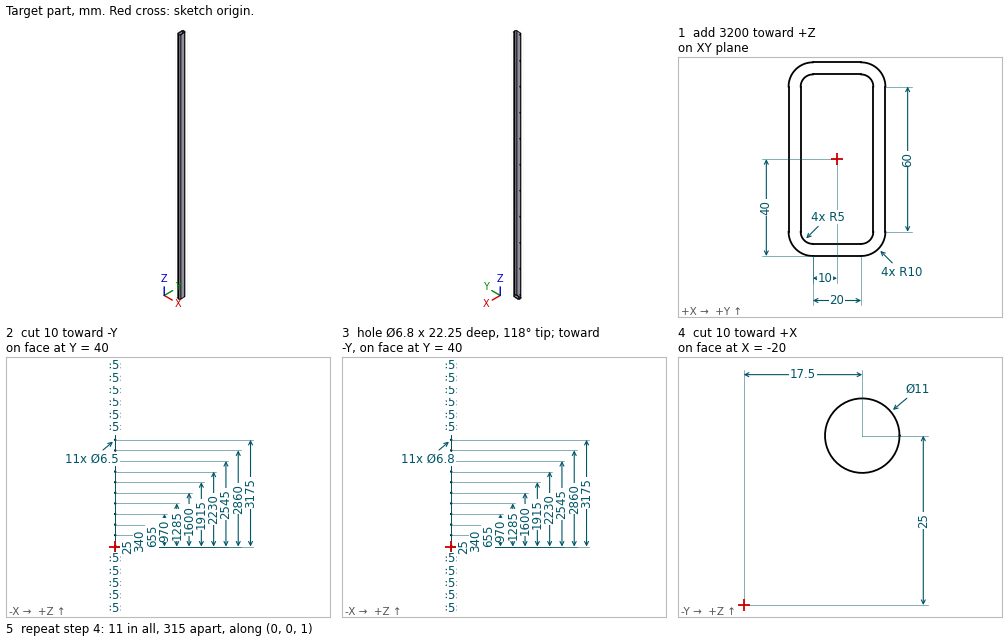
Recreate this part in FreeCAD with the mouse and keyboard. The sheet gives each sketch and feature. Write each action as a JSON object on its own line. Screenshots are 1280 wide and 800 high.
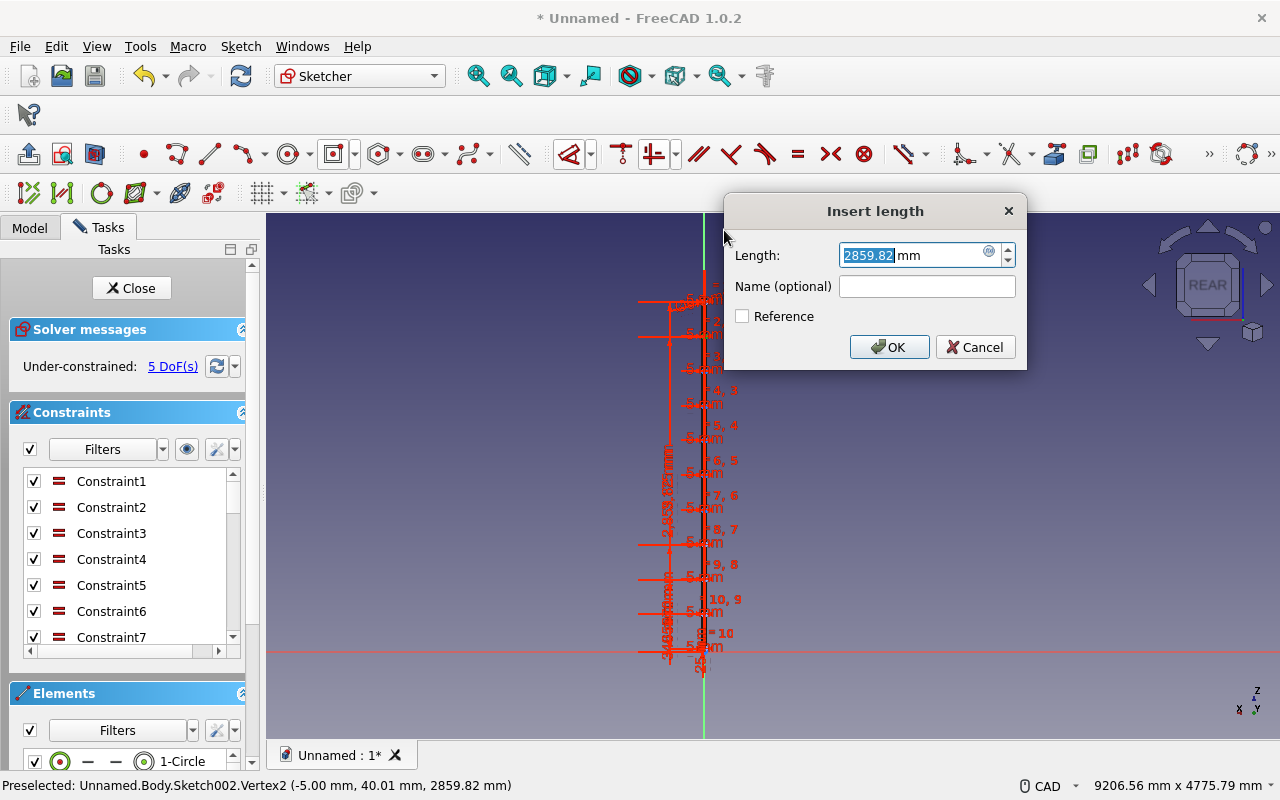
{"action": "type", "text": "2860"}
{"action": "key", "text": "Return"}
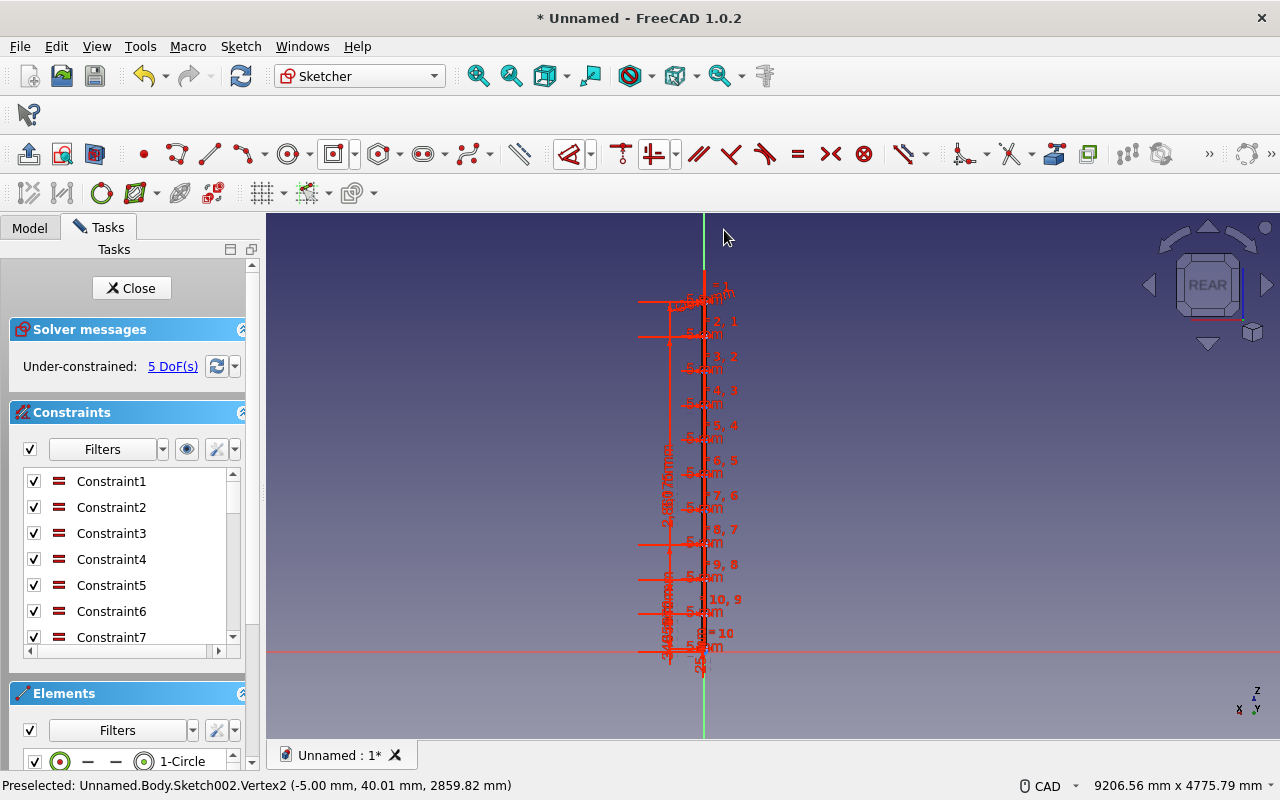
{"action": "left_click", "coordinate": [705, 371]}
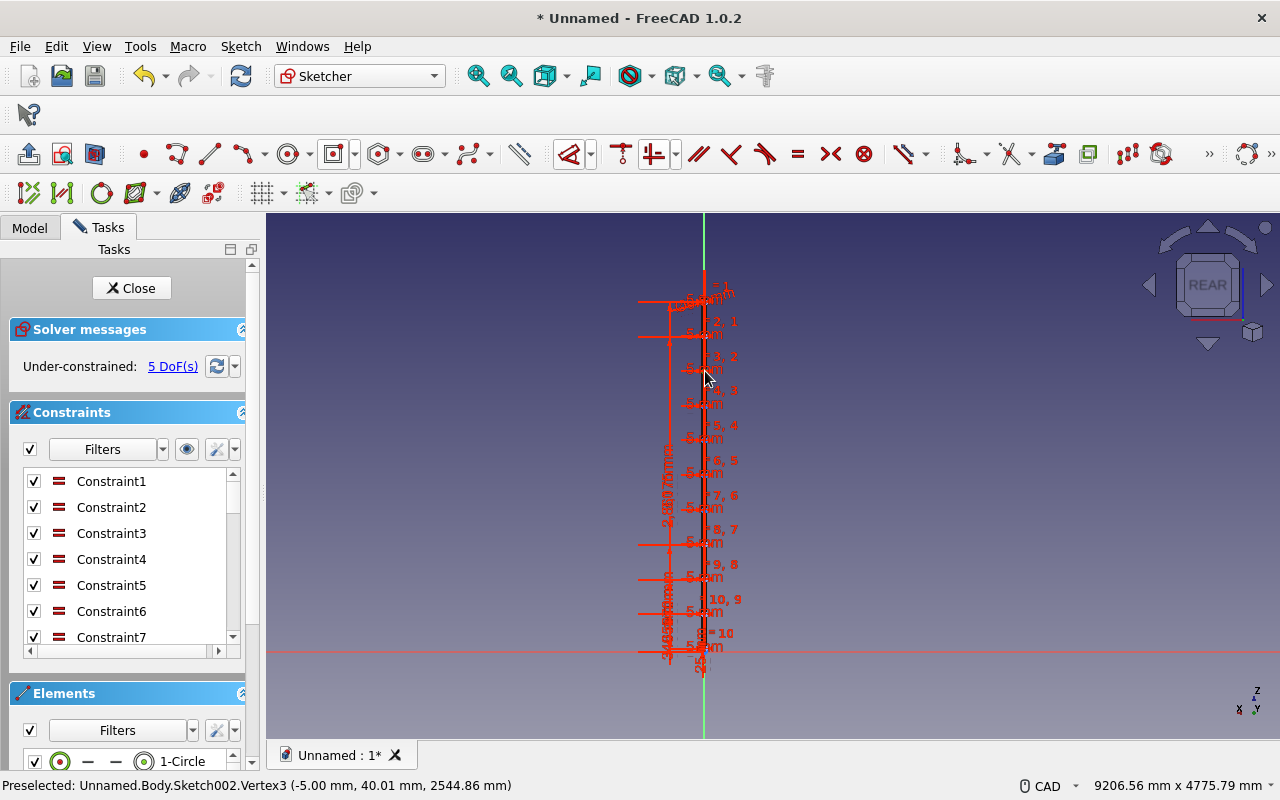
{"action": "left_click", "coordinate": [590, 154]}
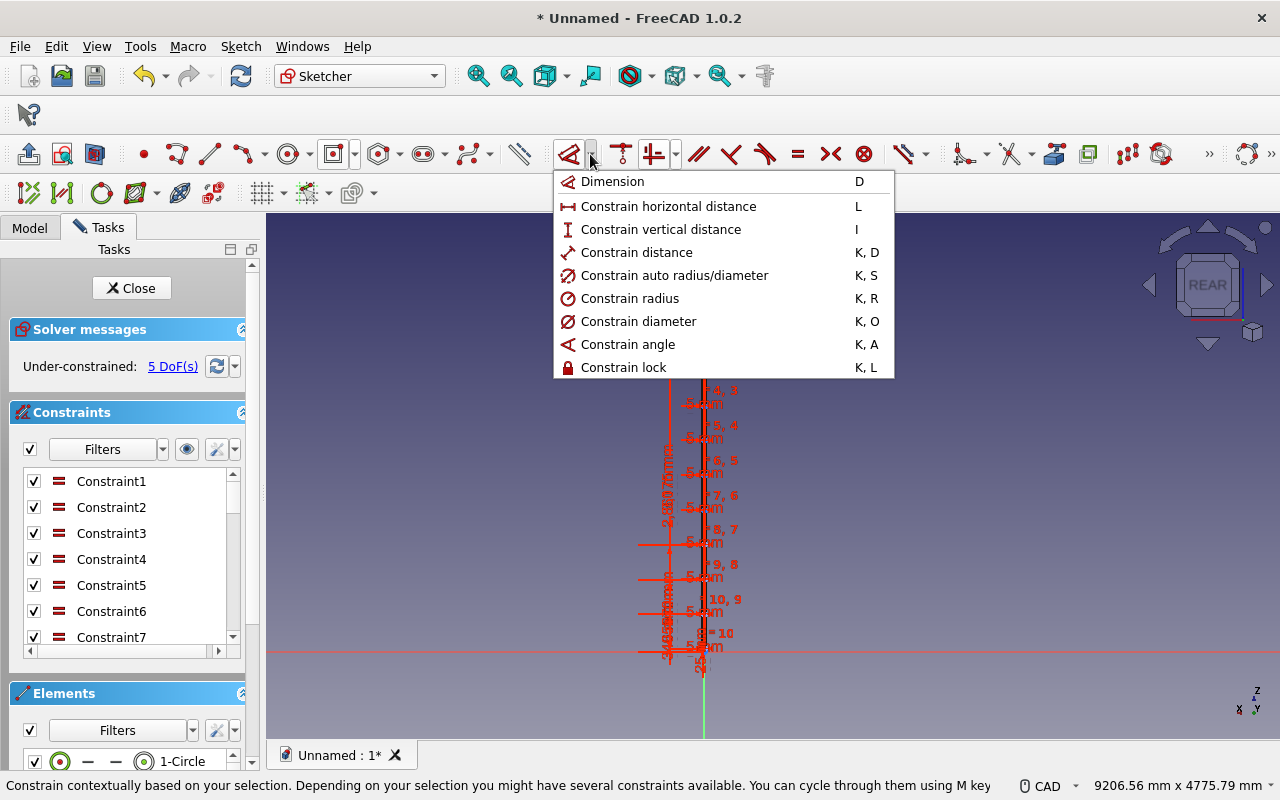
{"action": "left_click", "coordinate": [724, 230]}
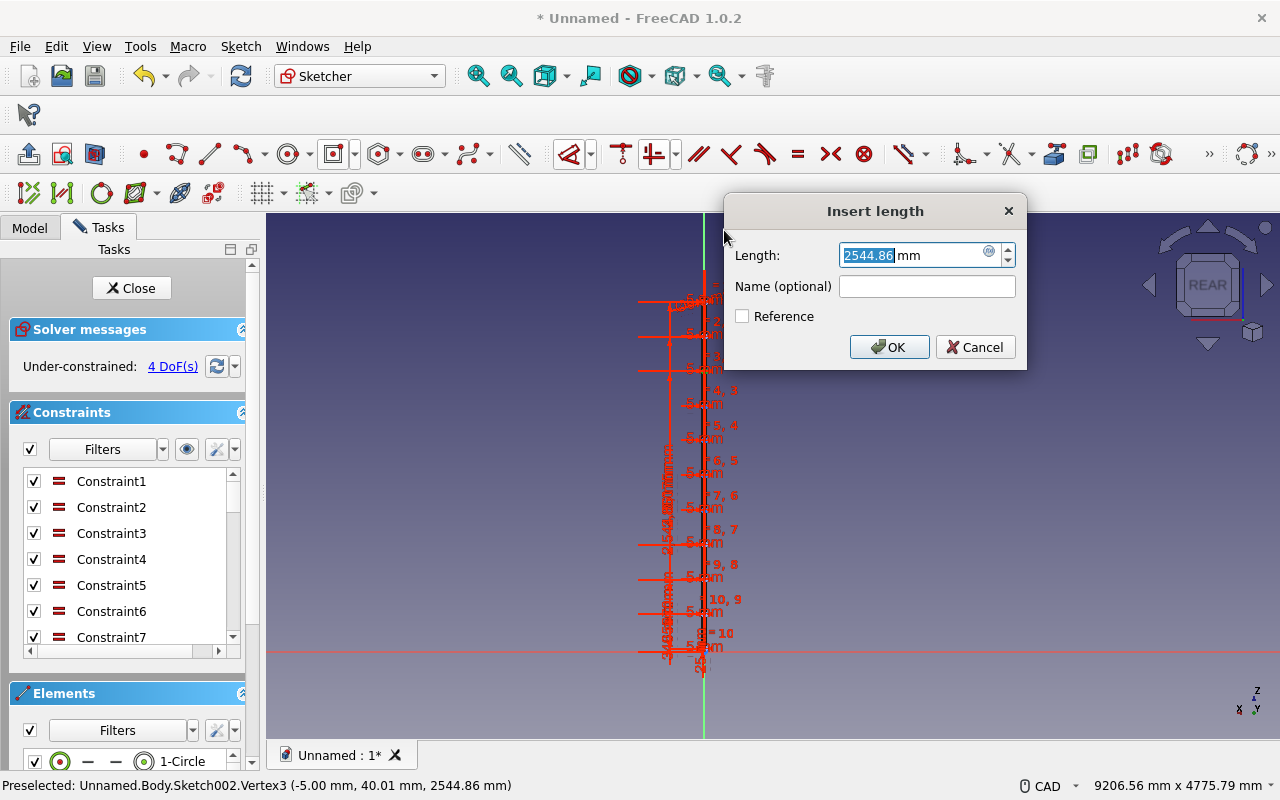
{"action": "type", "text": "2545"}
{"action": "key", "text": "Return"}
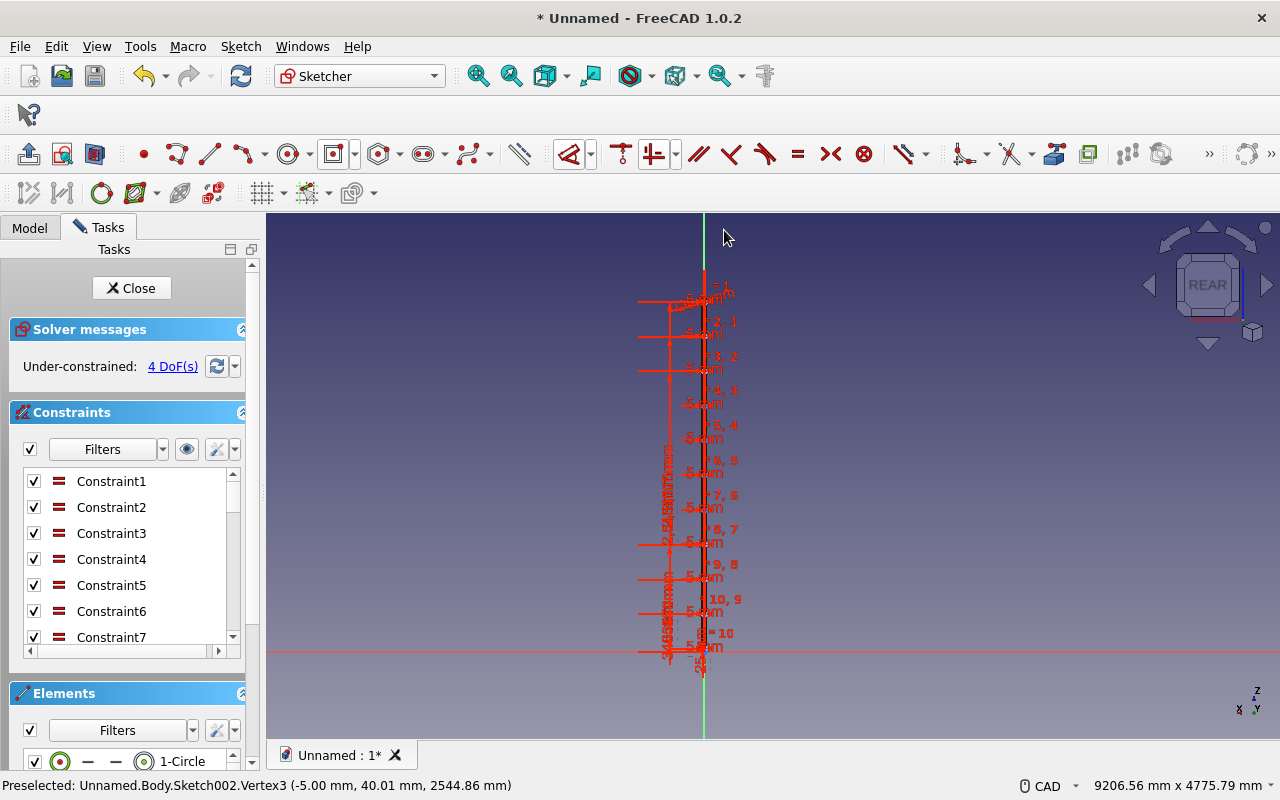
{"action": "left_click", "coordinate": [705, 406]}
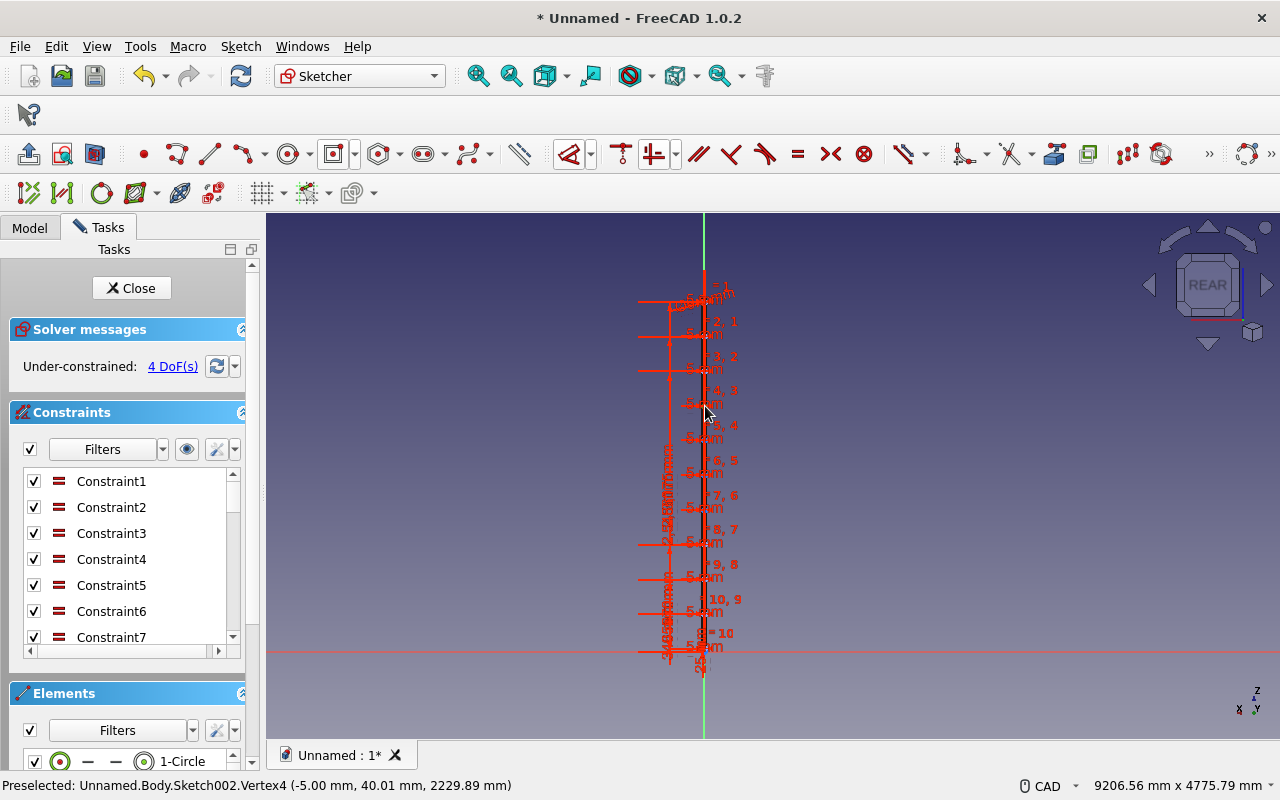
{"action": "key", "text": "i"}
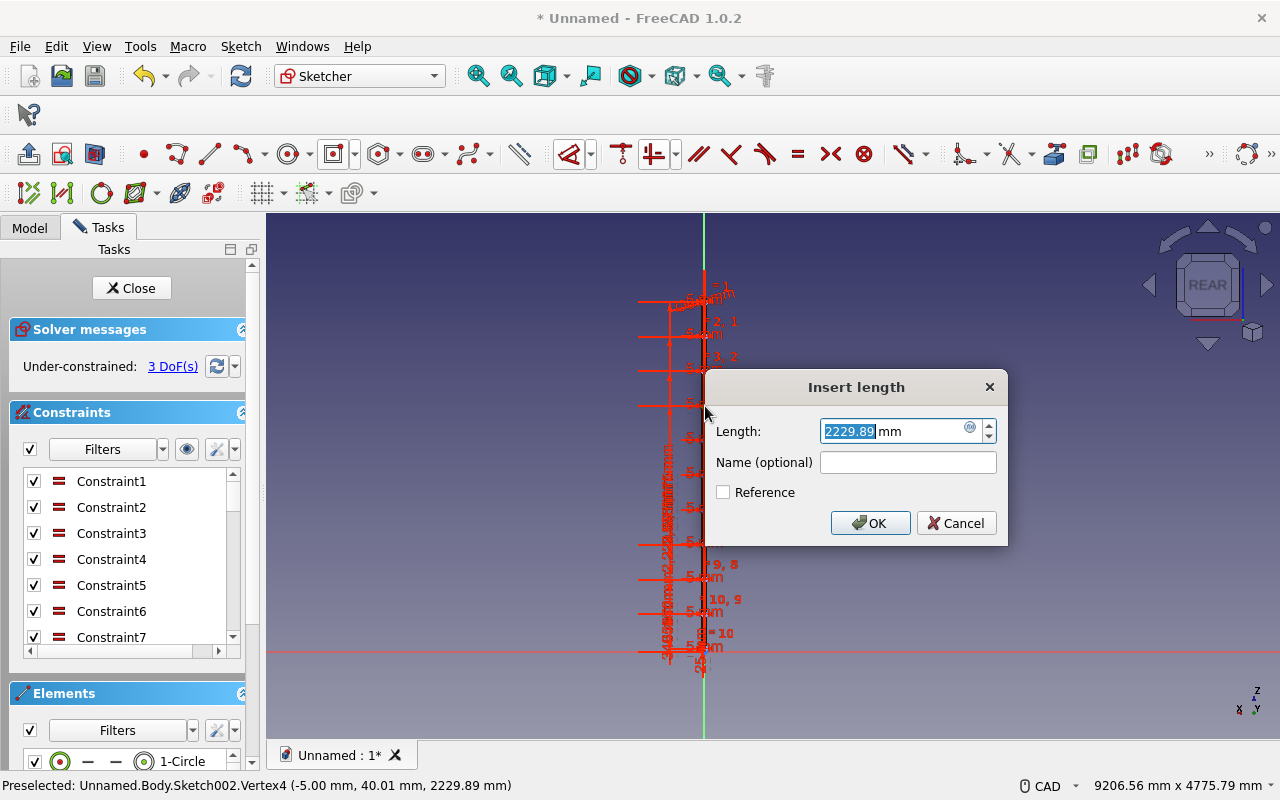
{"action": "type", "text": "2230"}
{"action": "key", "text": "Return"}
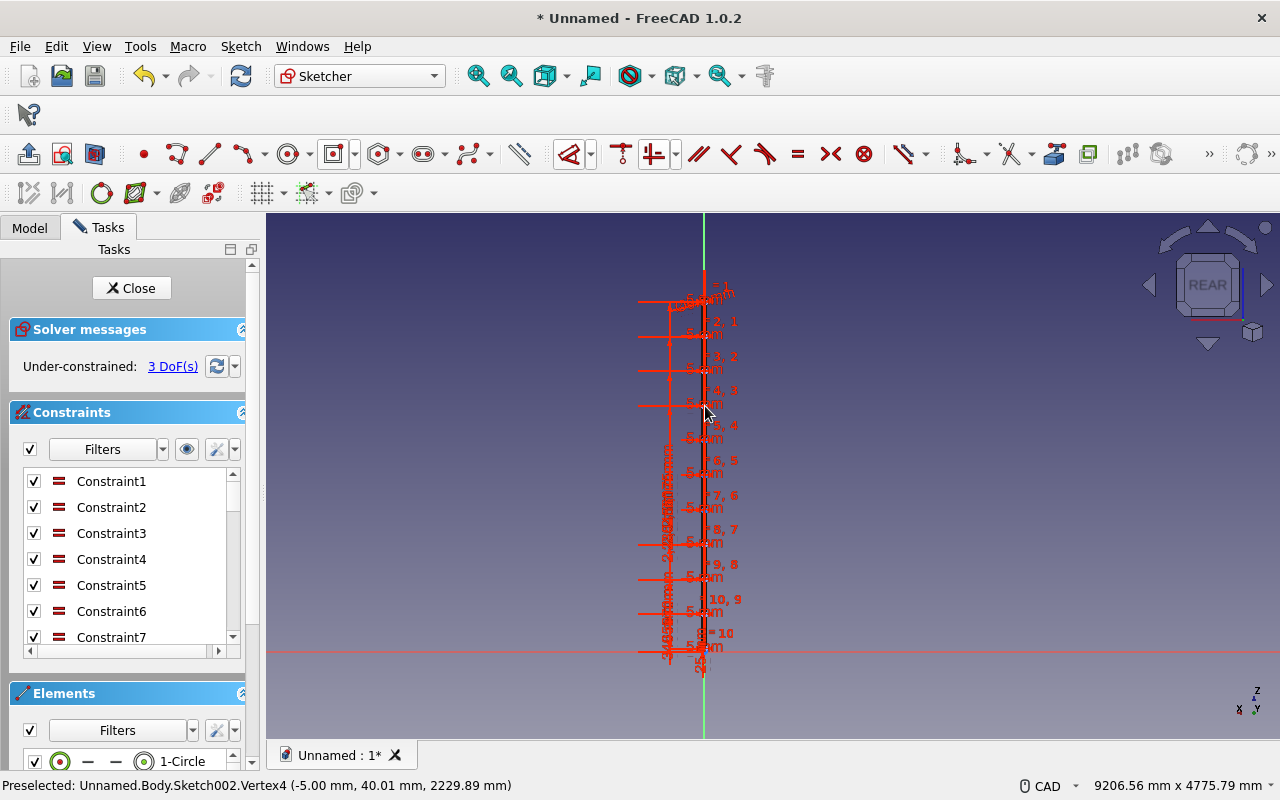
{"action": "left_click", "coordinate": [705, 441]}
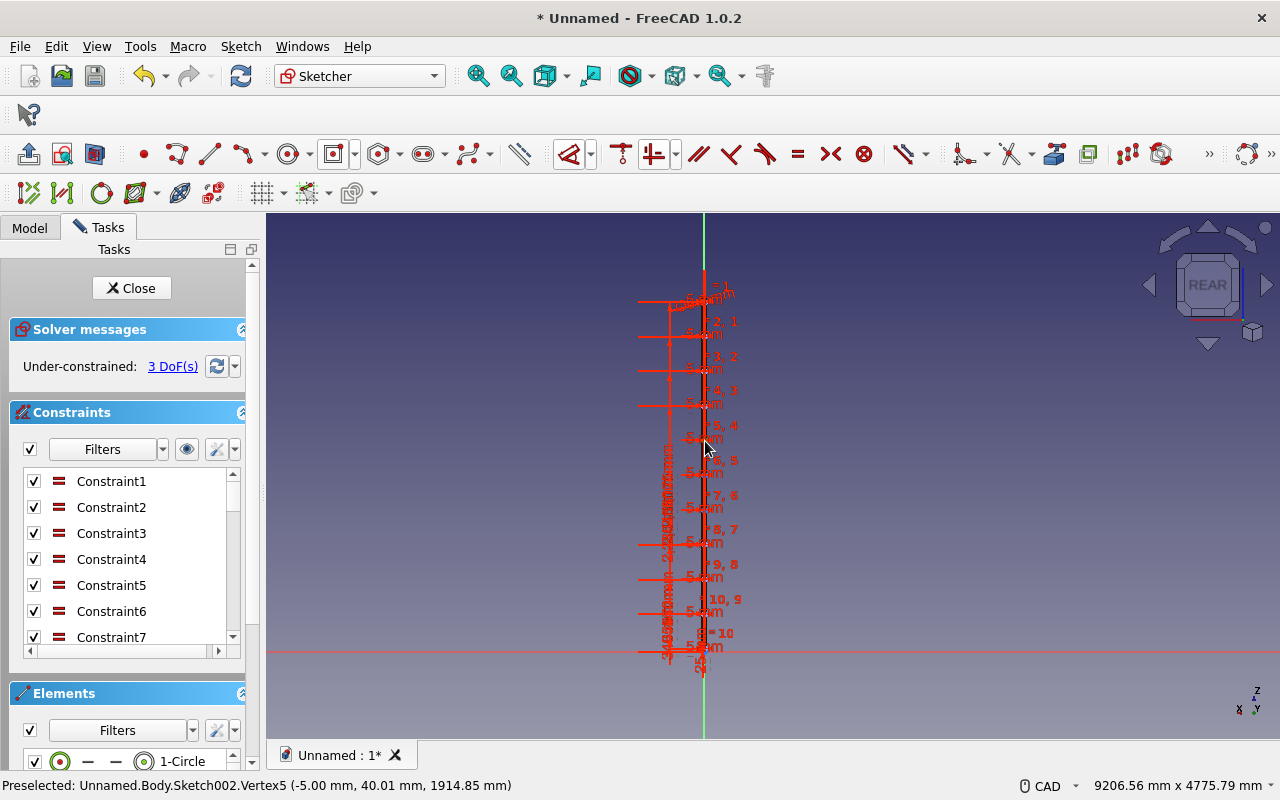
{"action": "left_click", "coordinate": [590, 154]}